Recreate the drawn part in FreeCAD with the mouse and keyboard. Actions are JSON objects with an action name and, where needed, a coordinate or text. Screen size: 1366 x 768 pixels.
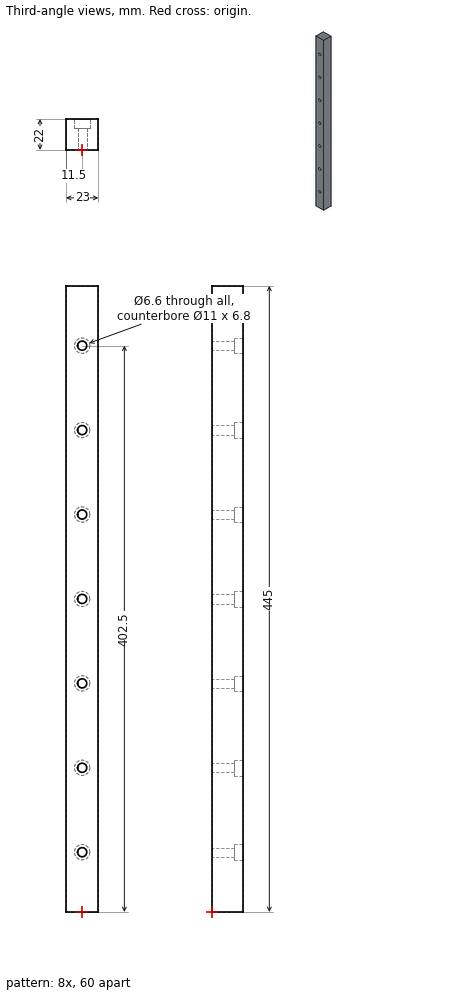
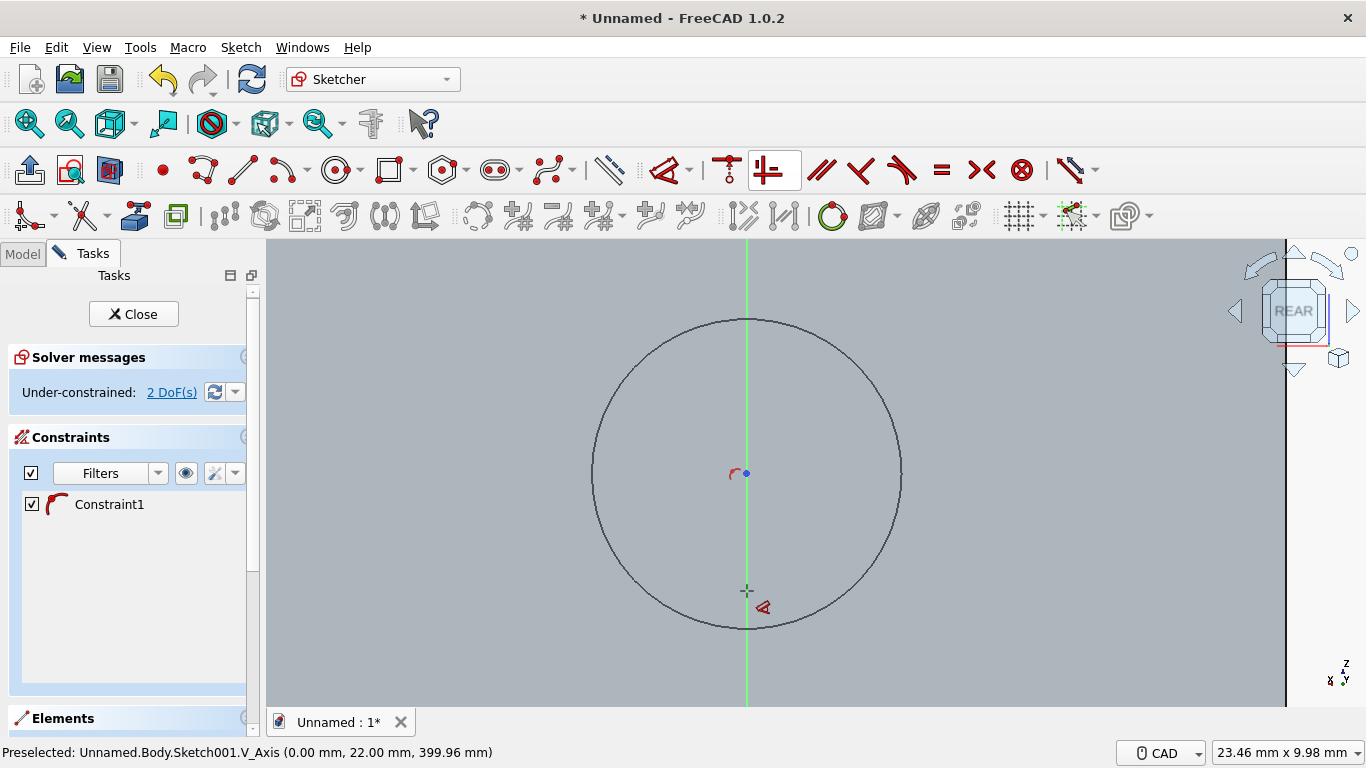
{"action": "left_click", "coordinate": [856, 364]}
{"action": "left_click", "coordinate": [879, 341]}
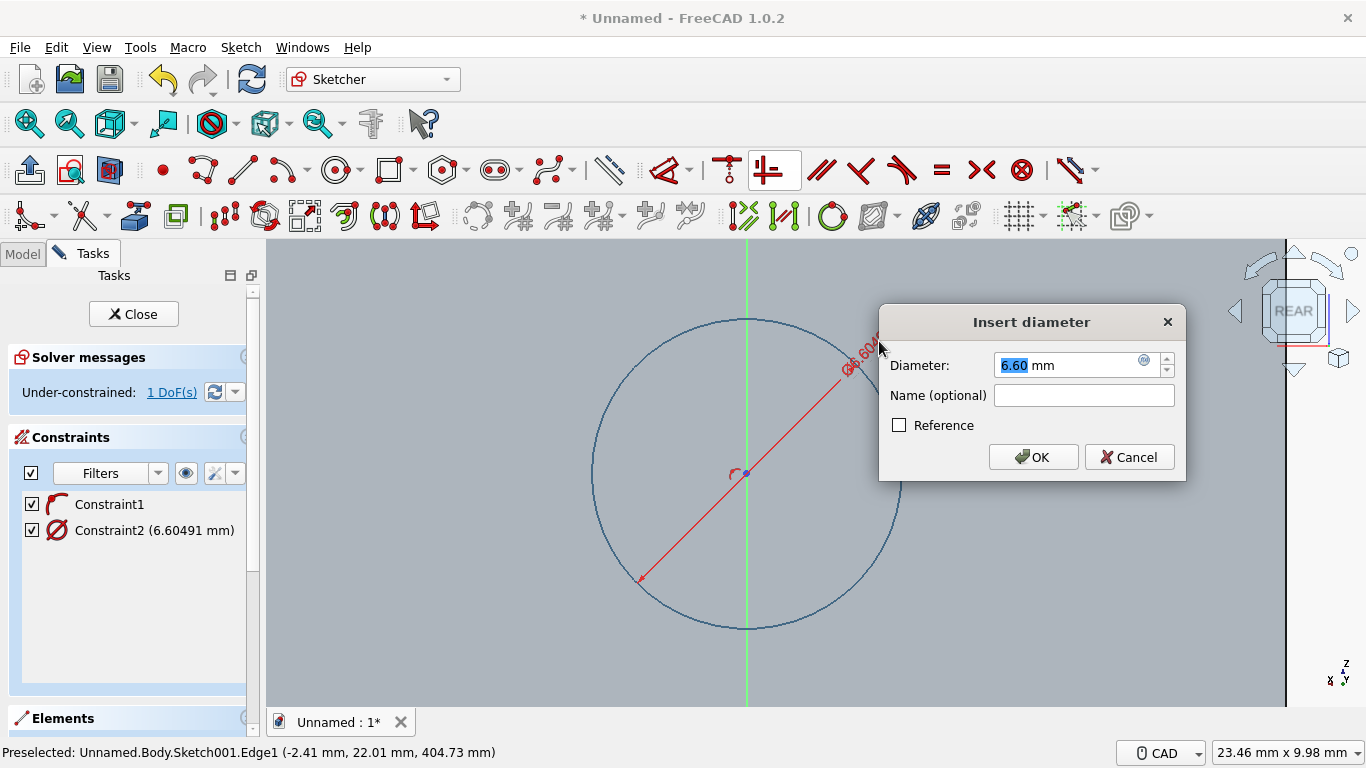
{"action": "type", "text": "6.6"}
{"action": "key", "text": "Return"}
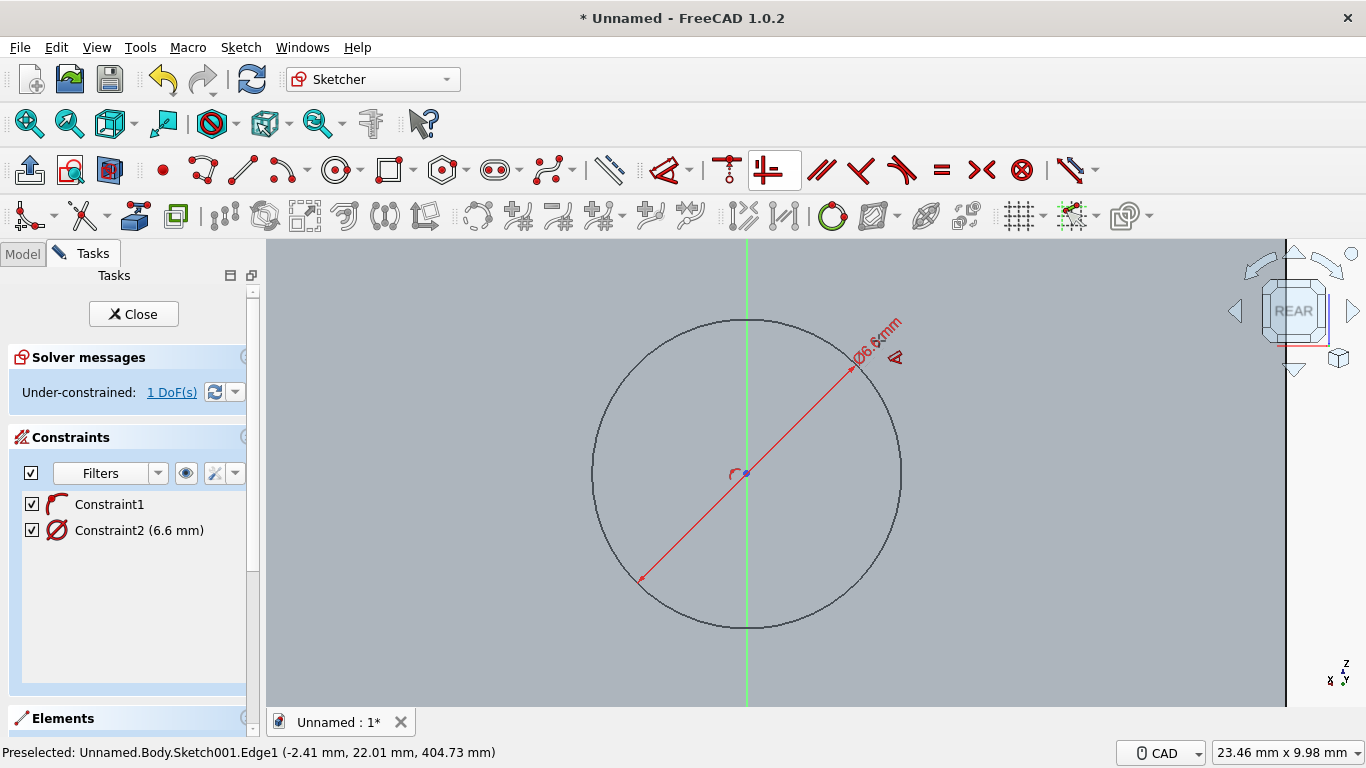
{"action": "left_click", "coordinate": [747, 474]}
{"action": "left_click", "coordinate": [781, 577]}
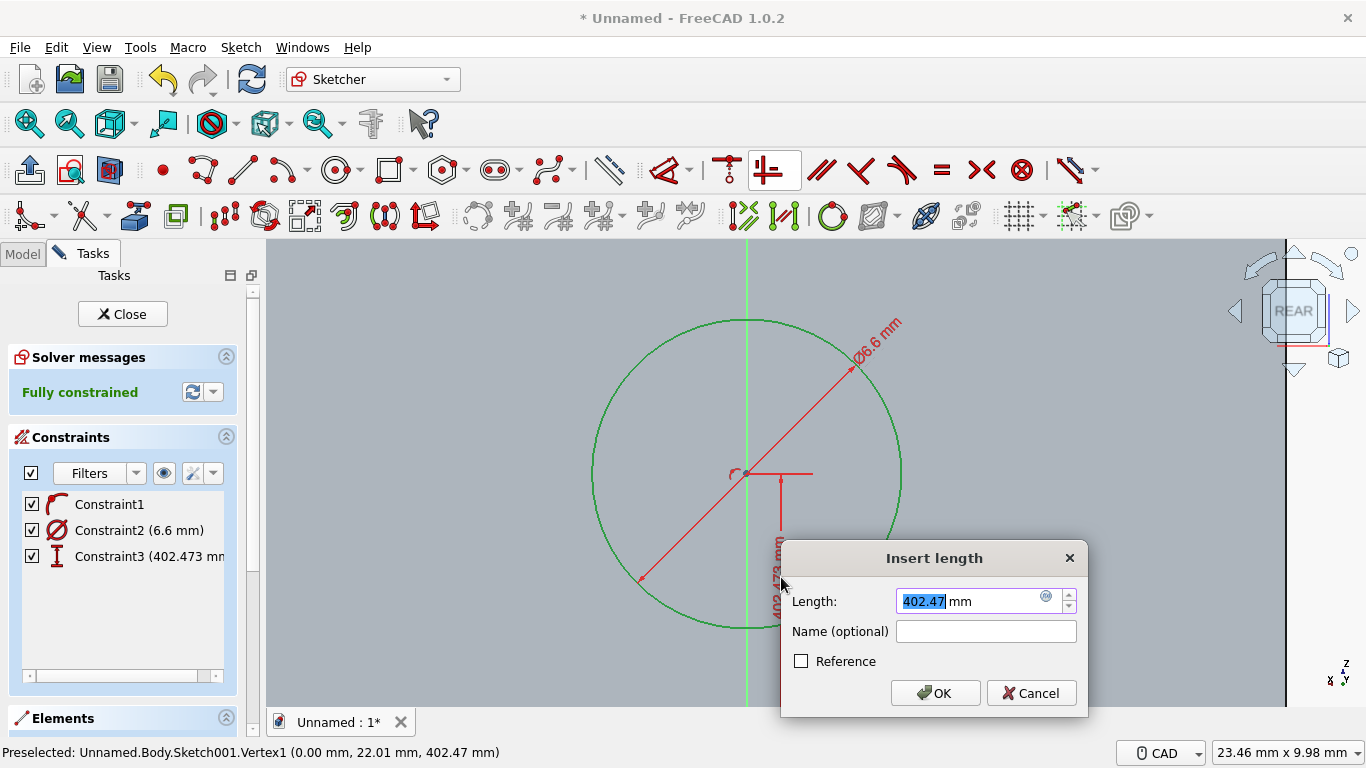
{"action": "type", "text": "402.5"}
{"action": "key", "text": "Return"}
{"action": "key", "text": "Escape"}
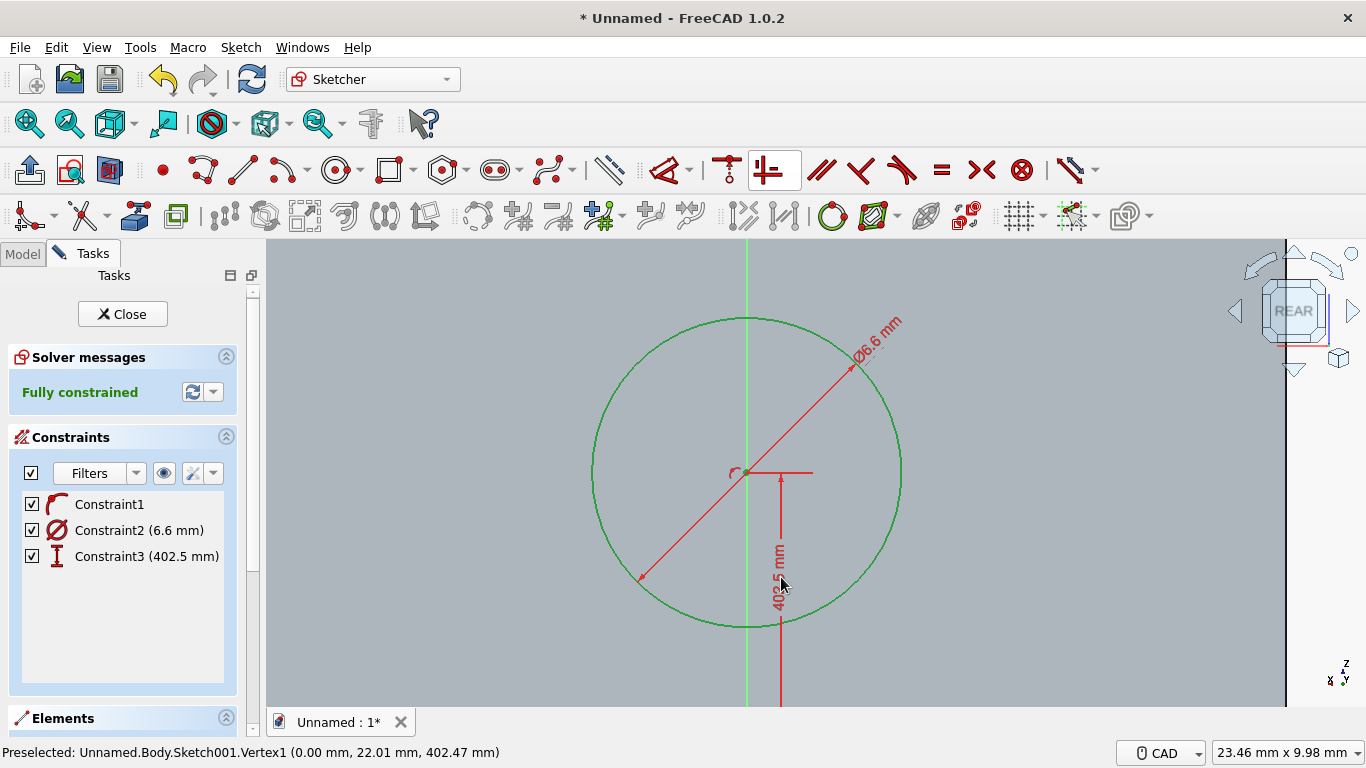
{"action": "left_click", "coordinate": [123, 314]}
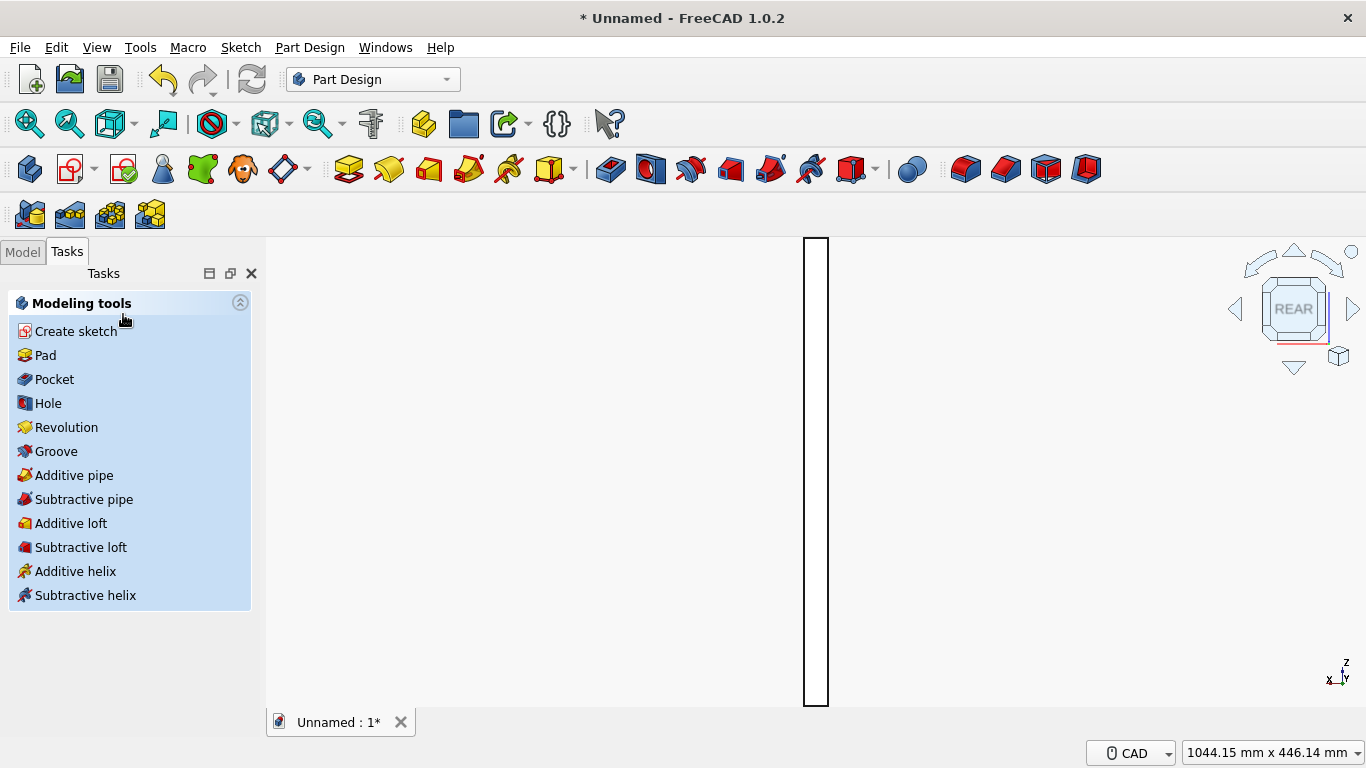
{"action": "left_click", "coordinate": [652, 170]}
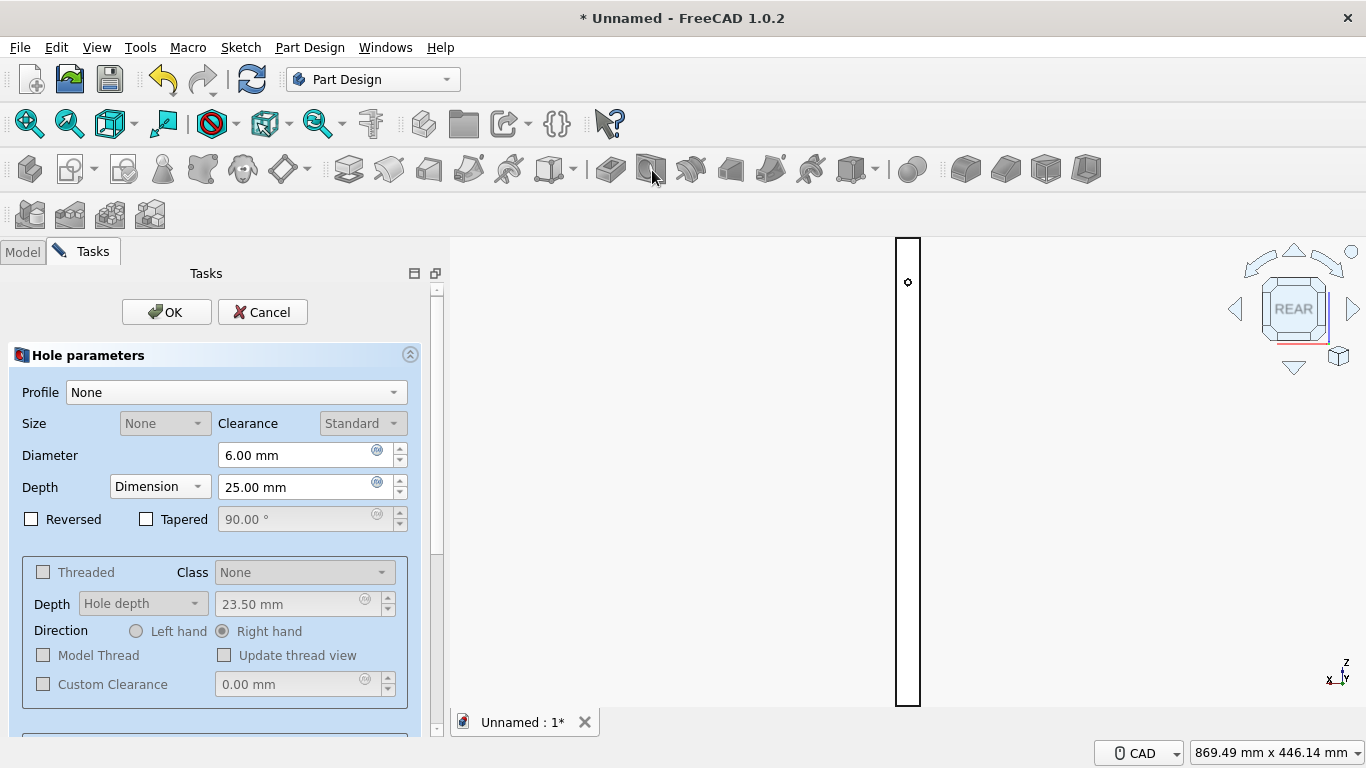
{"action": "triple_click", "coordinate": [305, 455]}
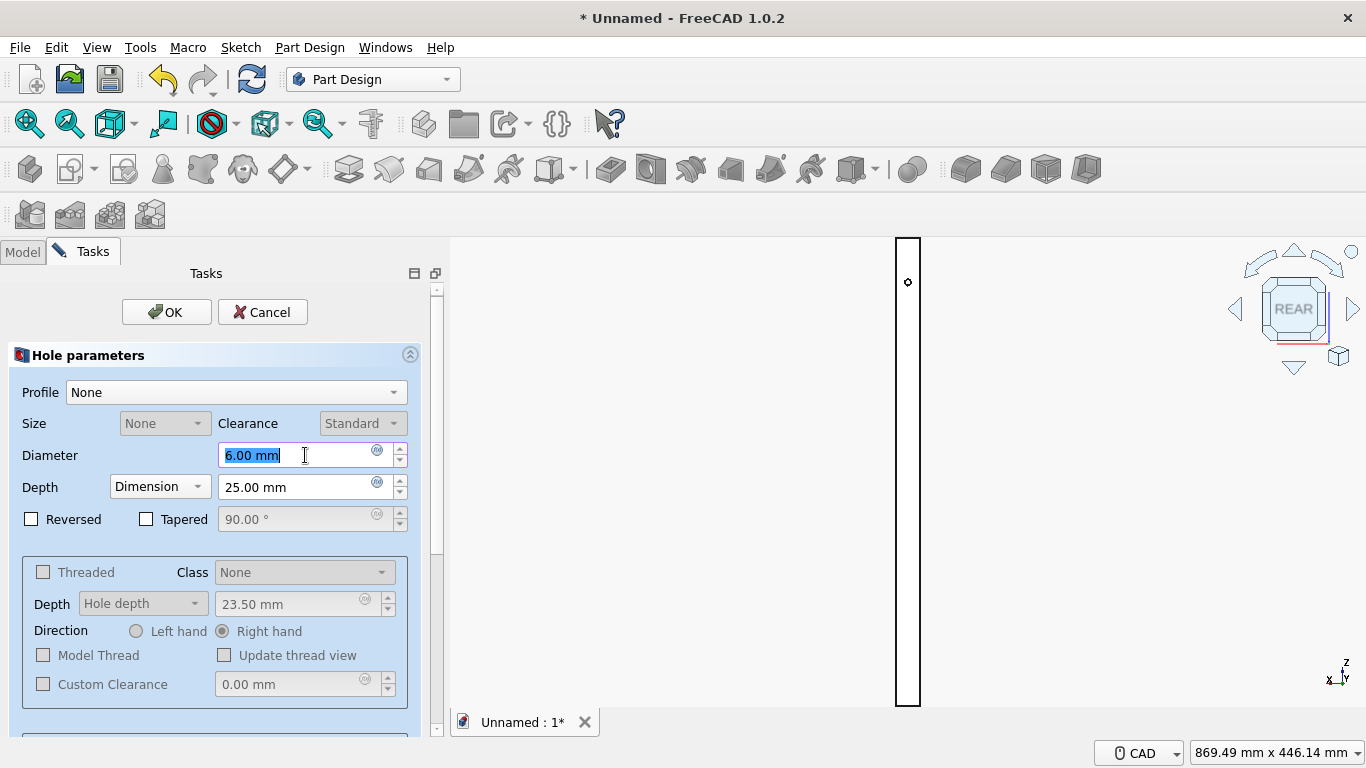
{"action": "type", "text": "6.6"}
{"action": "key", "text": "Tab"}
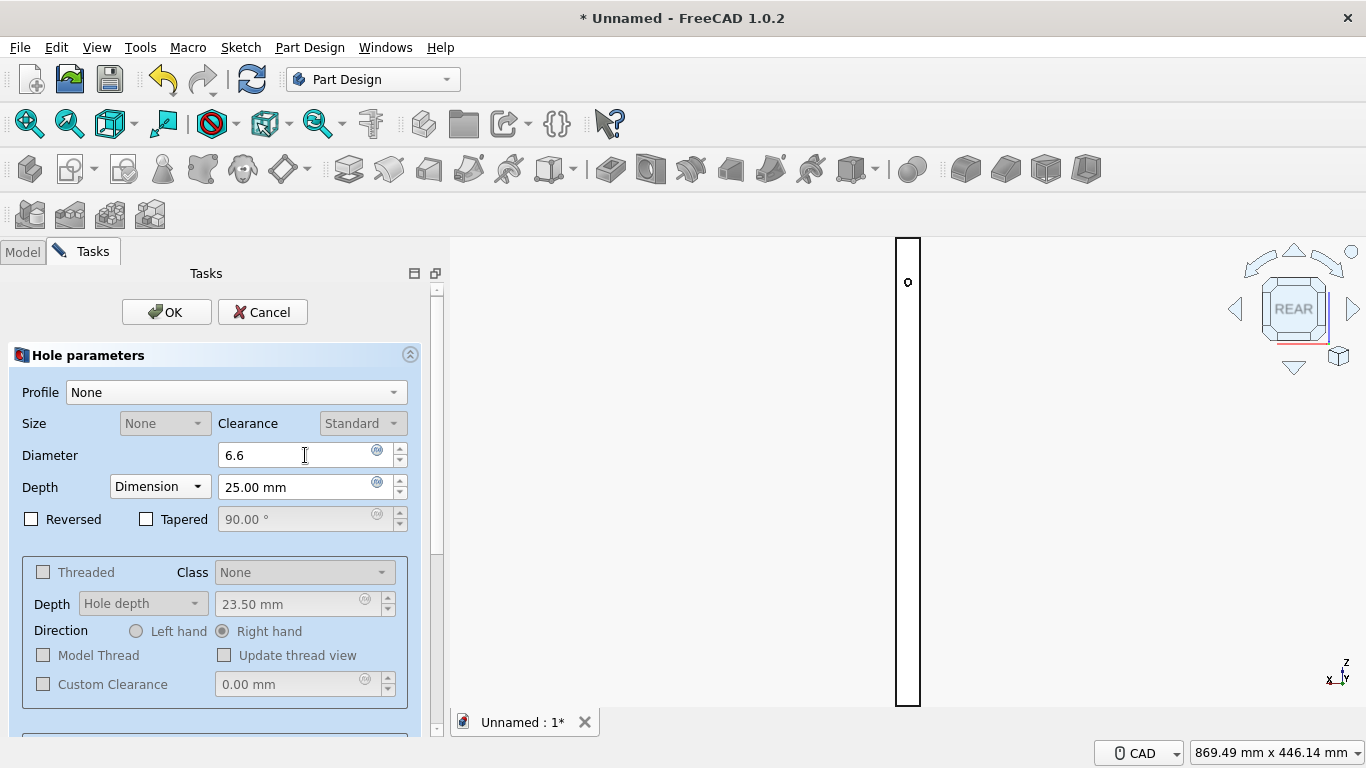
{"action": "left_click", "coordinate": [161, 486]}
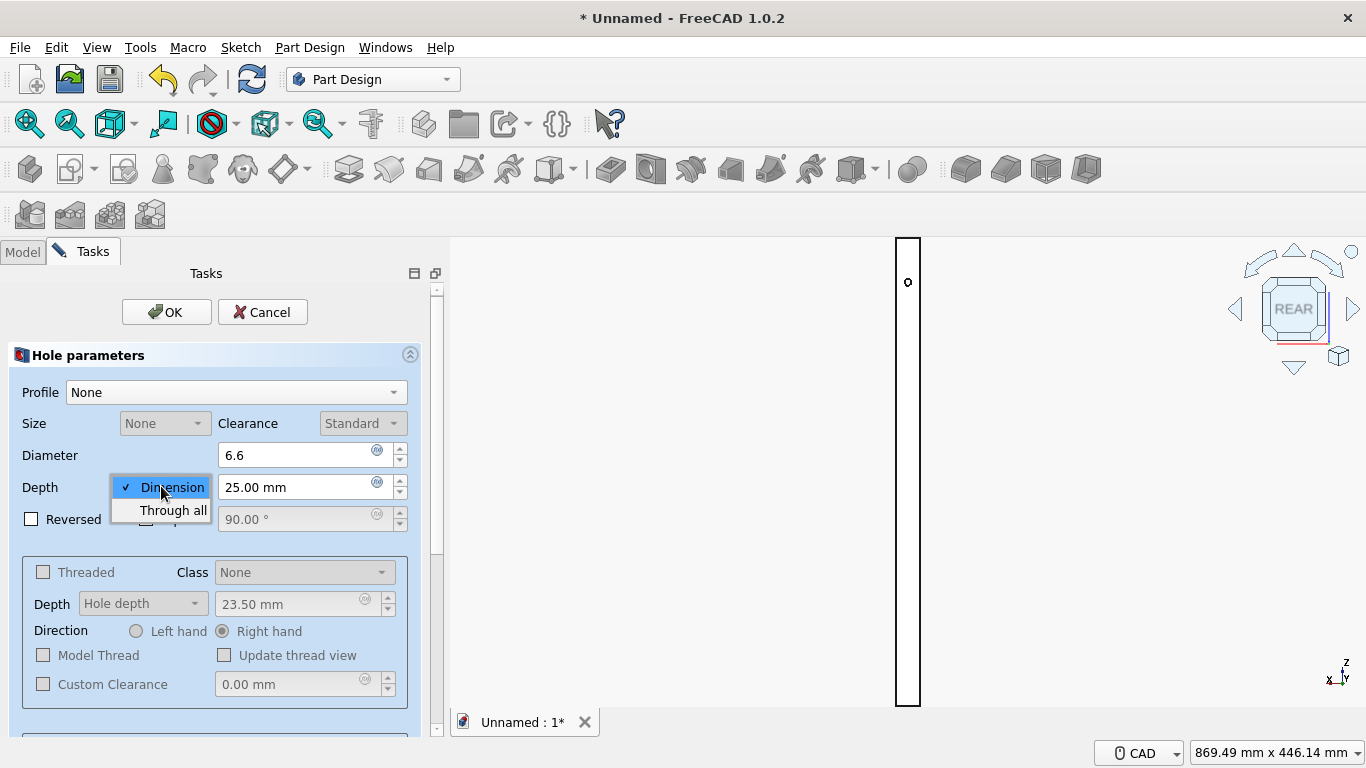
{"action": "left_click", "coordinate": [160, 510]}